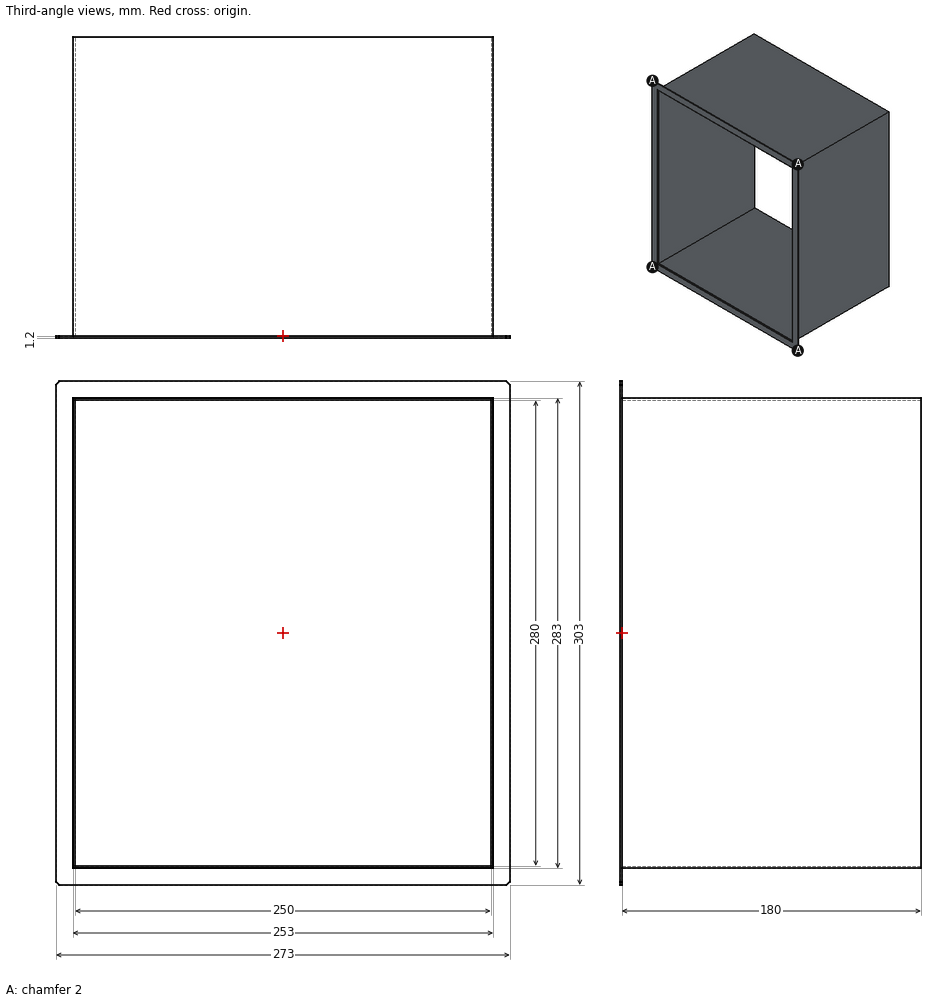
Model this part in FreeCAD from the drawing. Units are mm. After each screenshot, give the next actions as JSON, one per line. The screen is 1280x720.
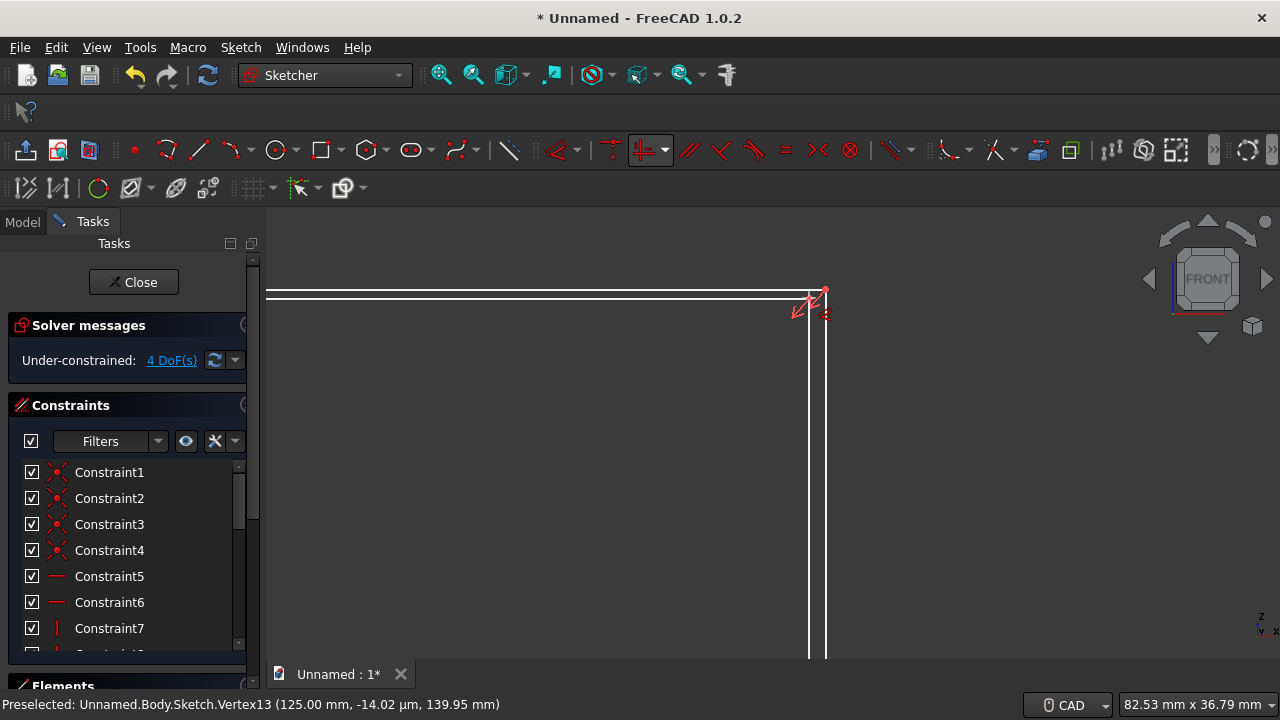
{"action": "scroll", "coordinate": [819, 306], "scroll_direction": "down", "scroll_amount": 13}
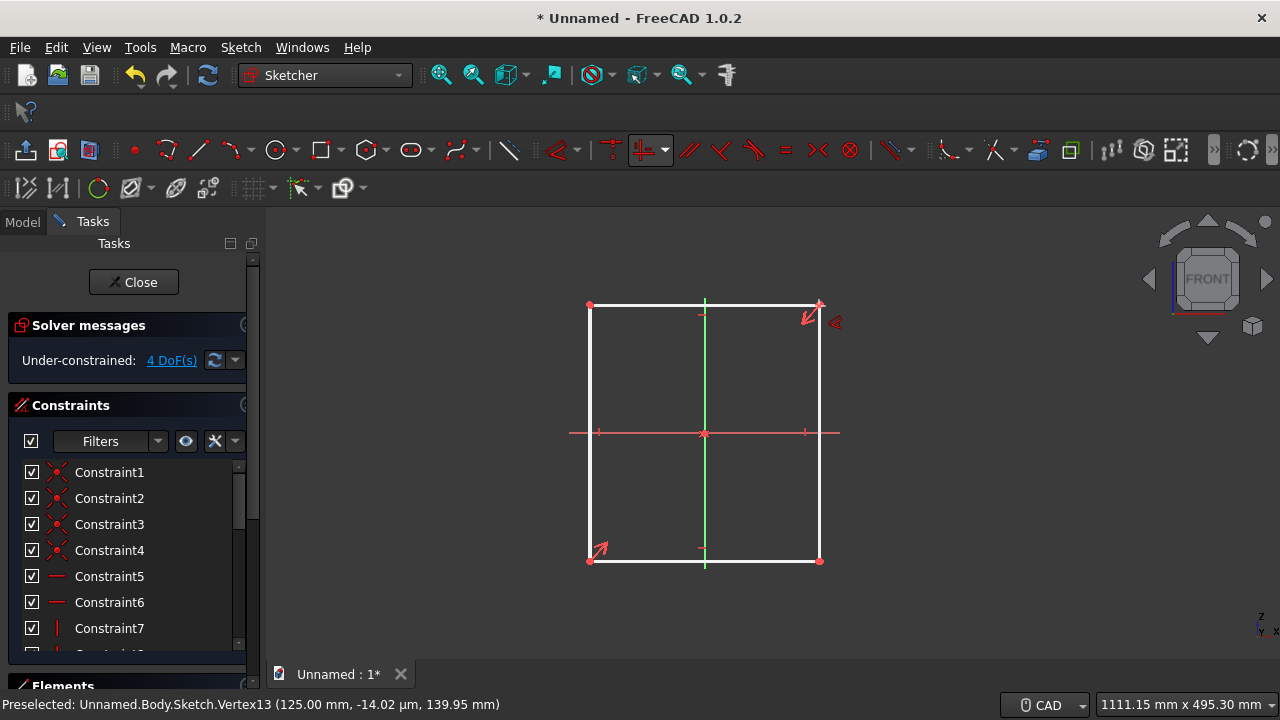
{"action": "scroll", "coordinate": [659, 562], "scroll_direction": "up", "scroll_amount": 14}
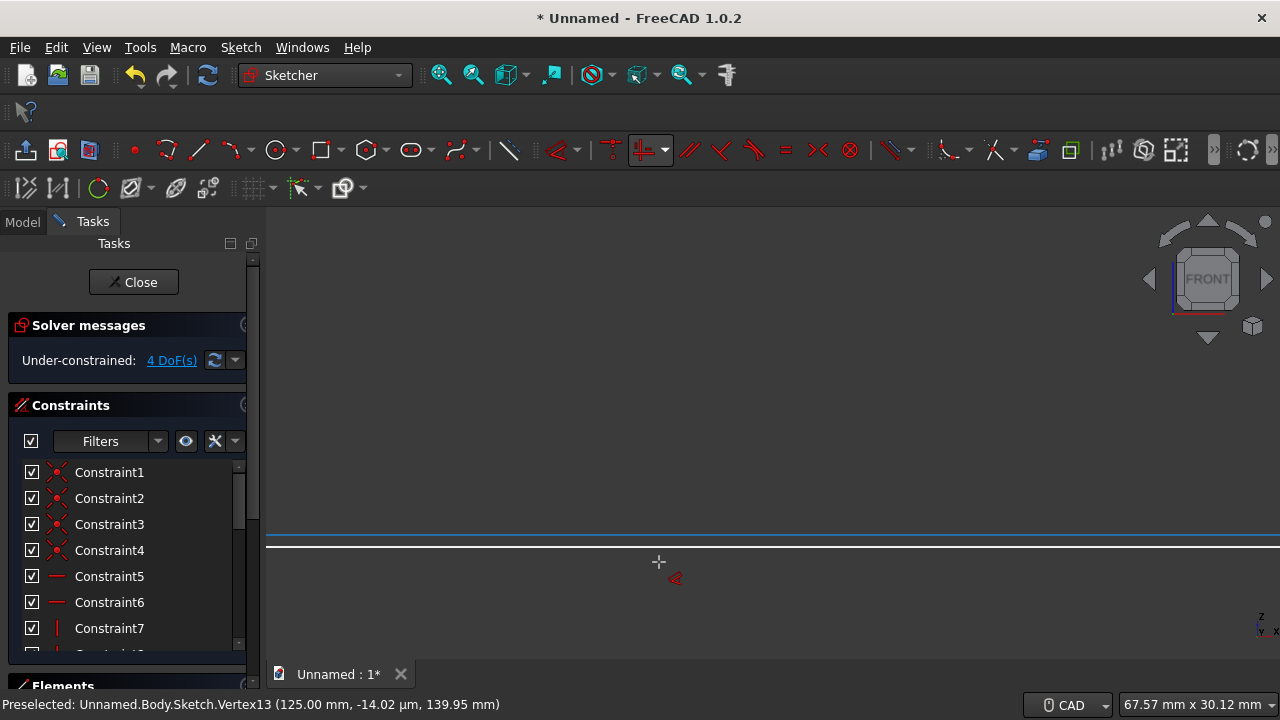
{"action": "left_click", "coordinate": [646, 547]}
{"action": "left_click", "coordinate": [704, 581]}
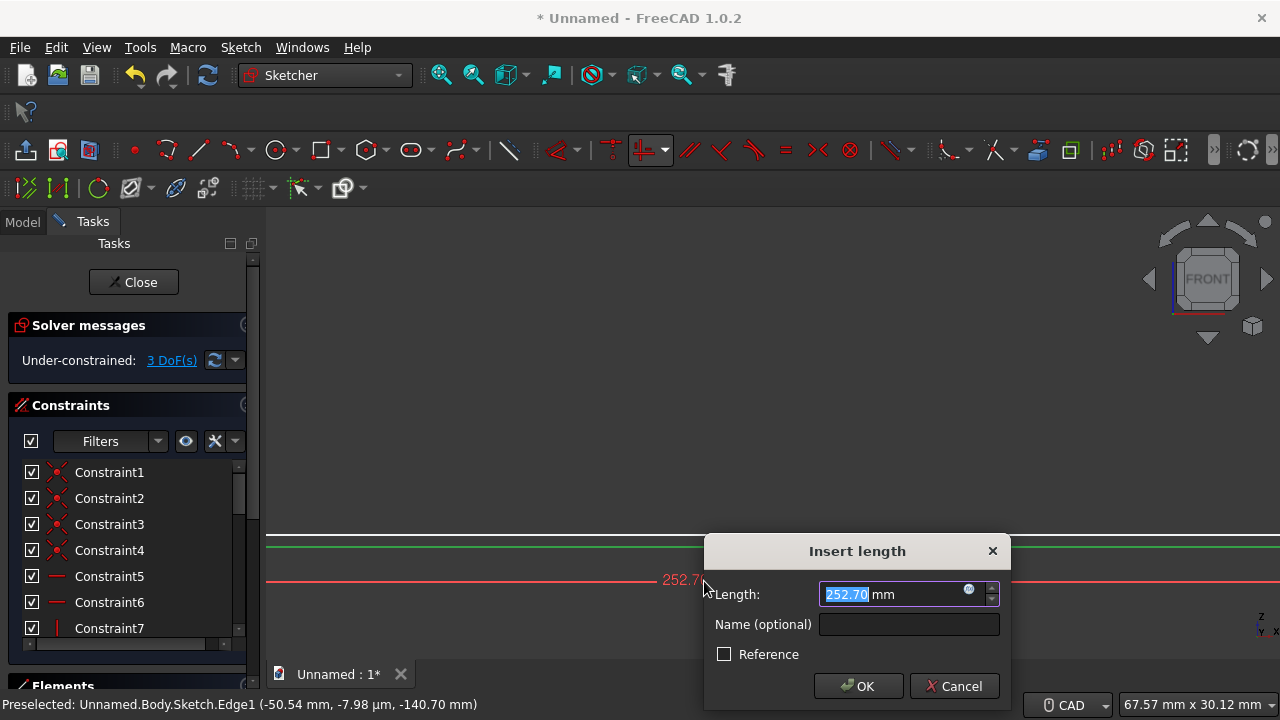
{"action": "type", "text": "253"}
{"action": "key", "text": "Return"}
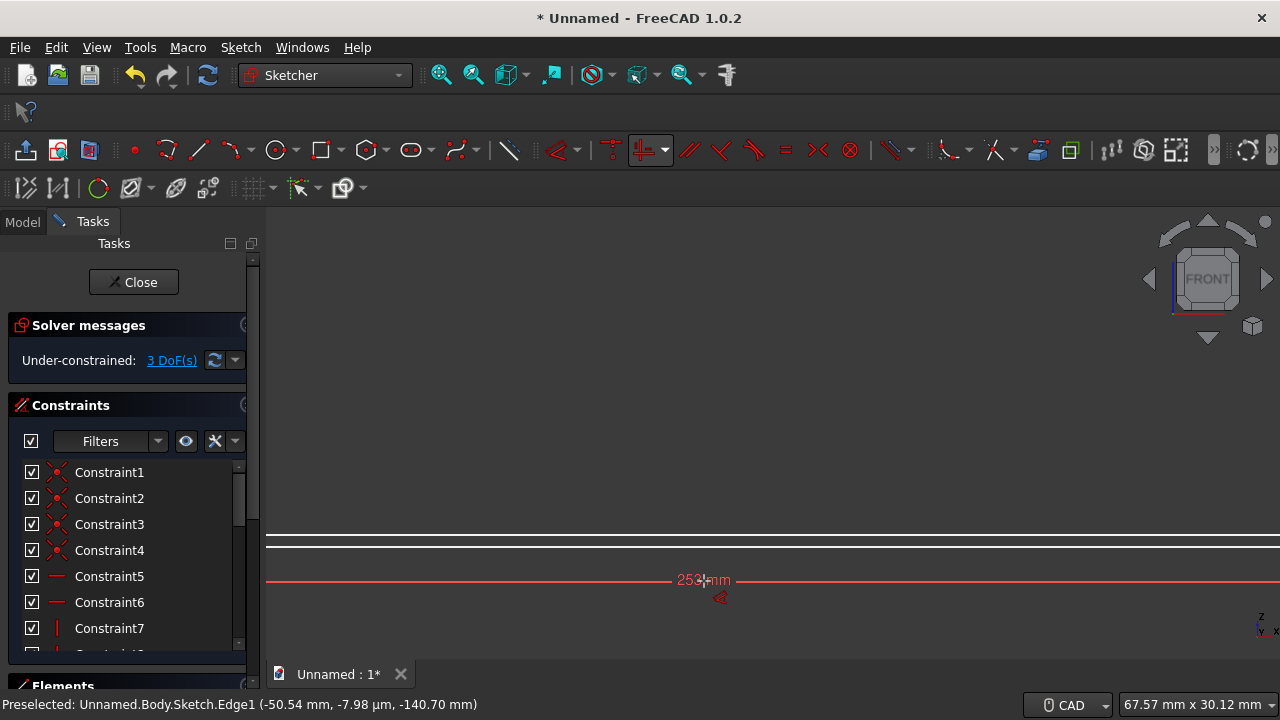
{"action": "scroll", "coordinate": [659, 562], "scroll_direction": "down", "scroll_amount": 14}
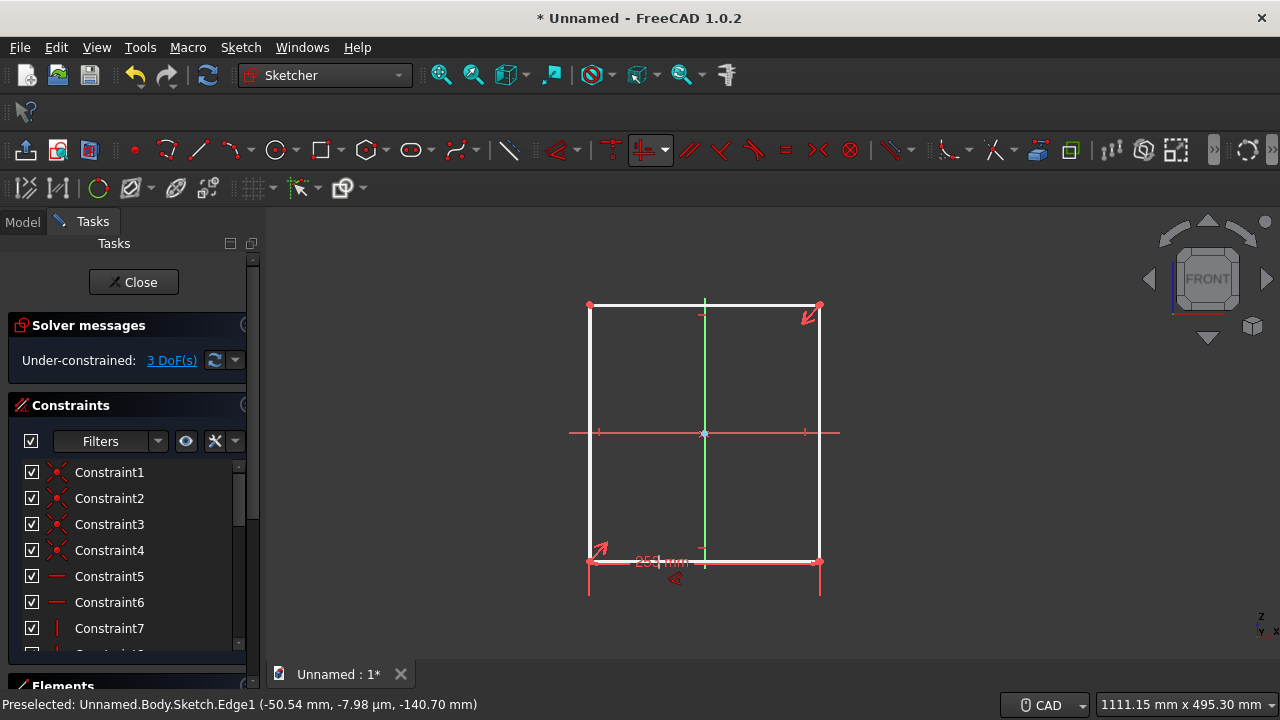
{"action": "scroll", "coordinate": [820, 485], "scroll_direction": "up", "scroll_amount": 12}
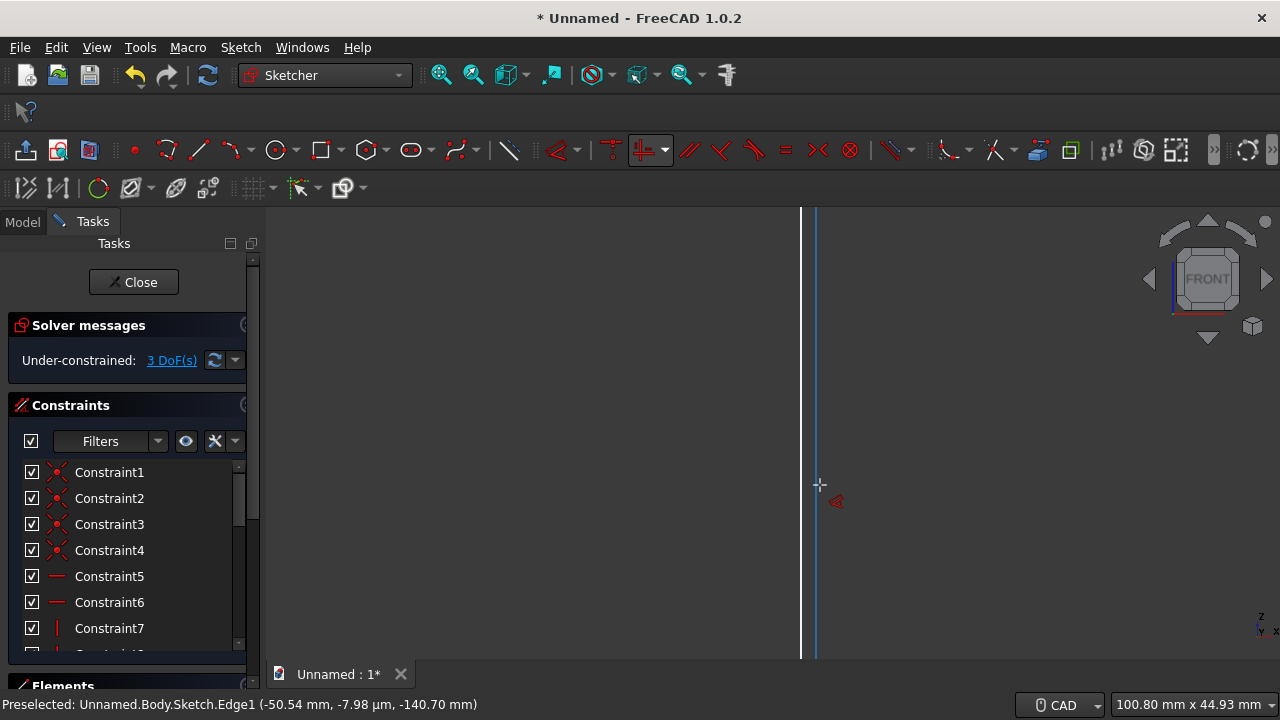
{"action": "left_click", "coordinate": [816, 476]}
{"action": "left_click", "coordinate": [850, 433]}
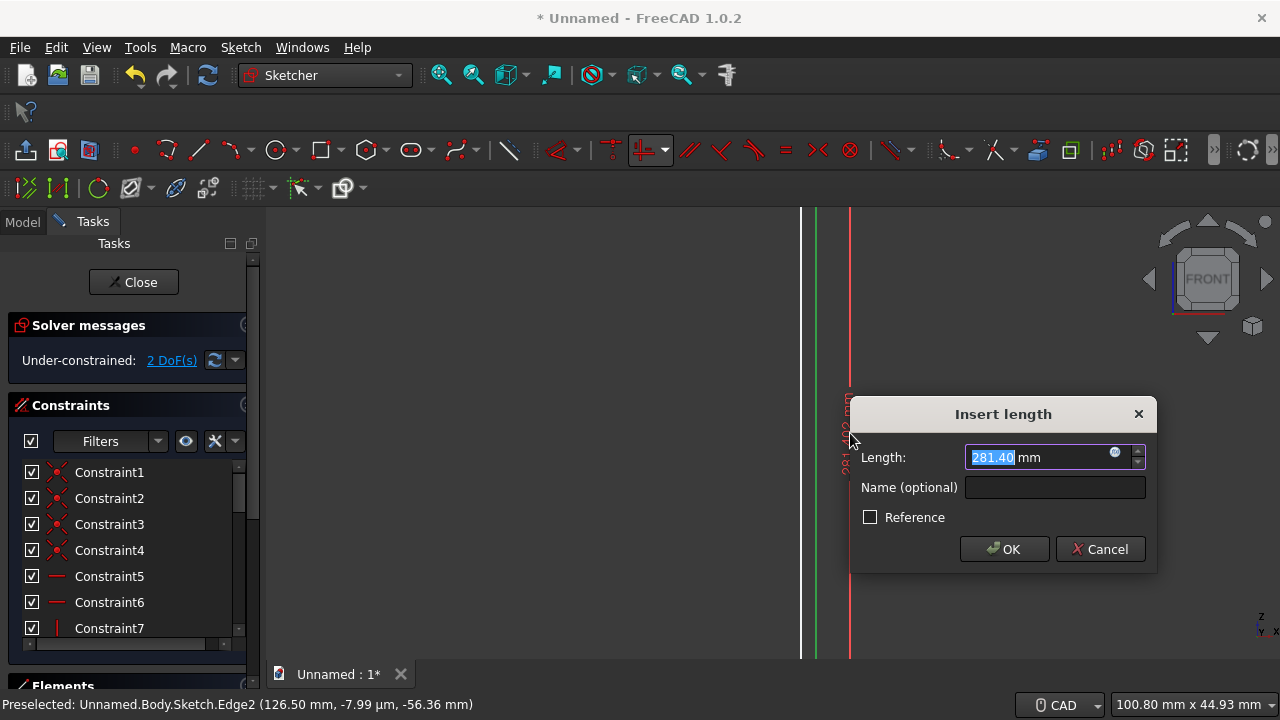
{"action": "type", "text": "283"}
{"action": "key", "text": "Return"}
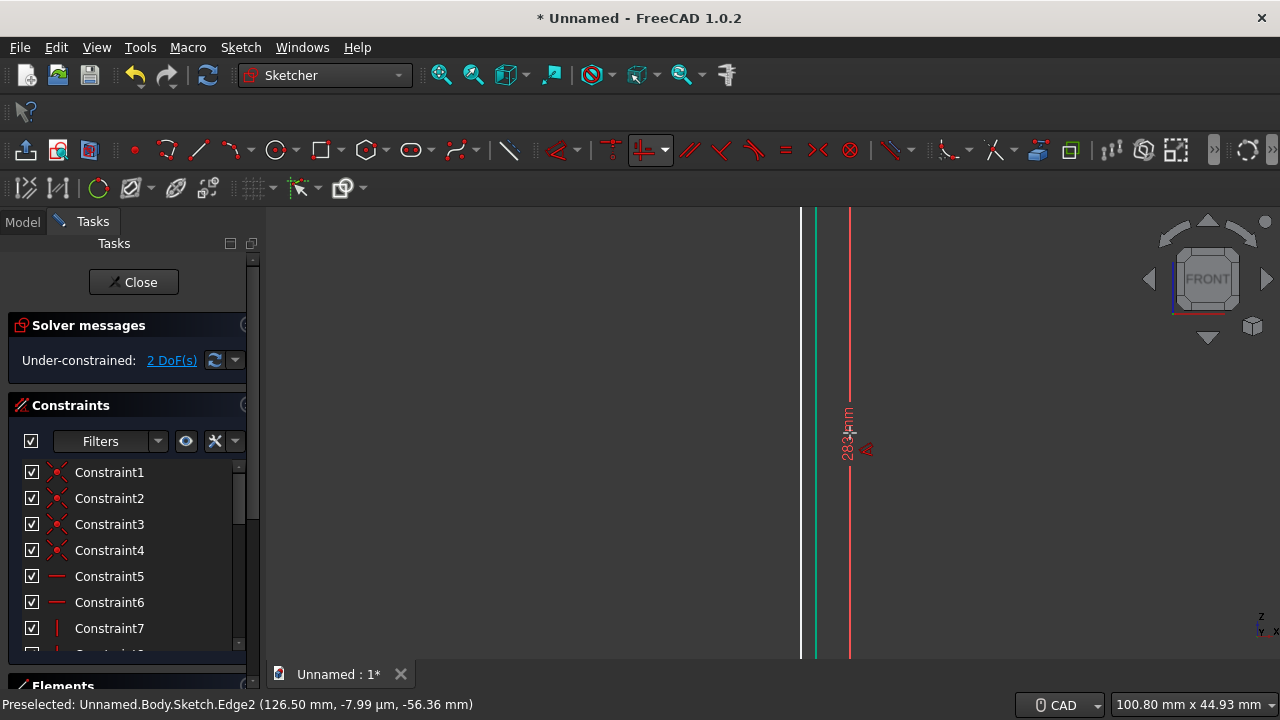
{"action": "scroll", "coordinate": [820, 485], "scroll_direction": "down", "scroll_amount": 12}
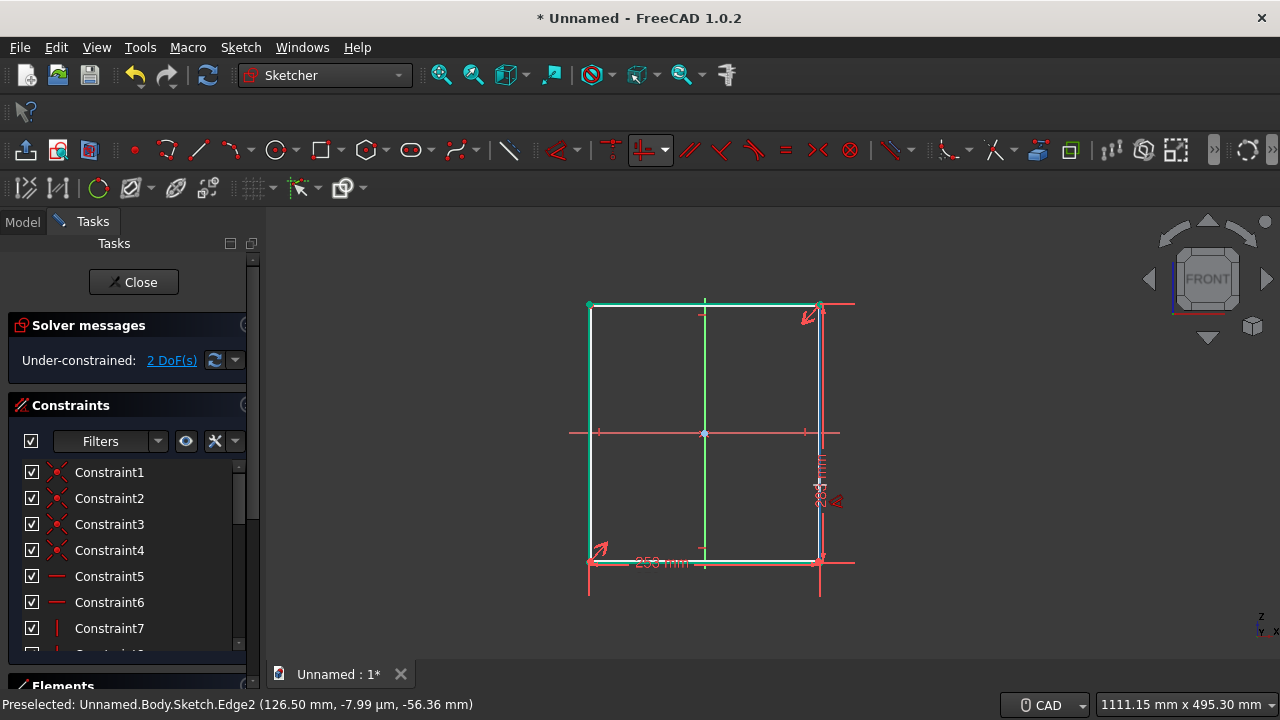
{"action": "scroll", "coordinate": [659, 561], "scroll_direction": "up", "scroll_amount": 12}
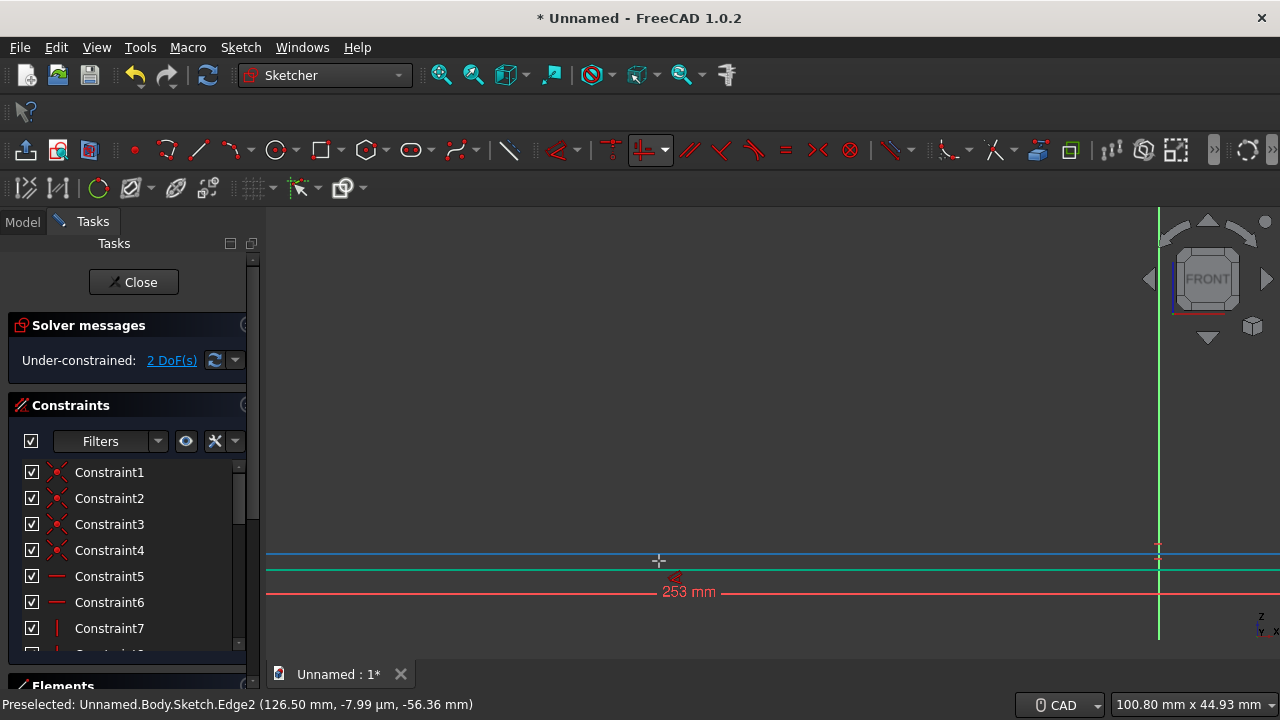
{"action": "left_click", "coordinate": [656, 554]}
{"action": "left_click", "coordinate": [516, 588]}